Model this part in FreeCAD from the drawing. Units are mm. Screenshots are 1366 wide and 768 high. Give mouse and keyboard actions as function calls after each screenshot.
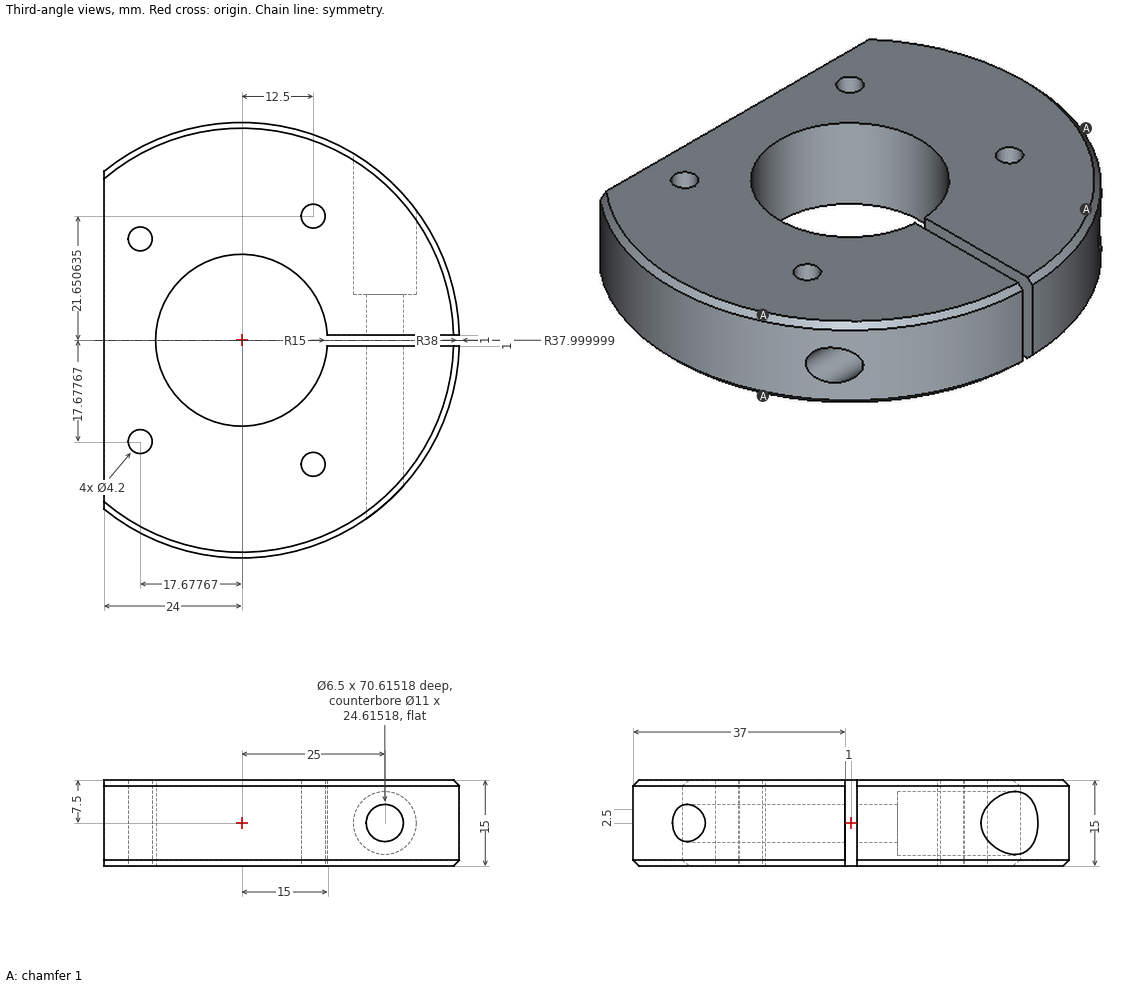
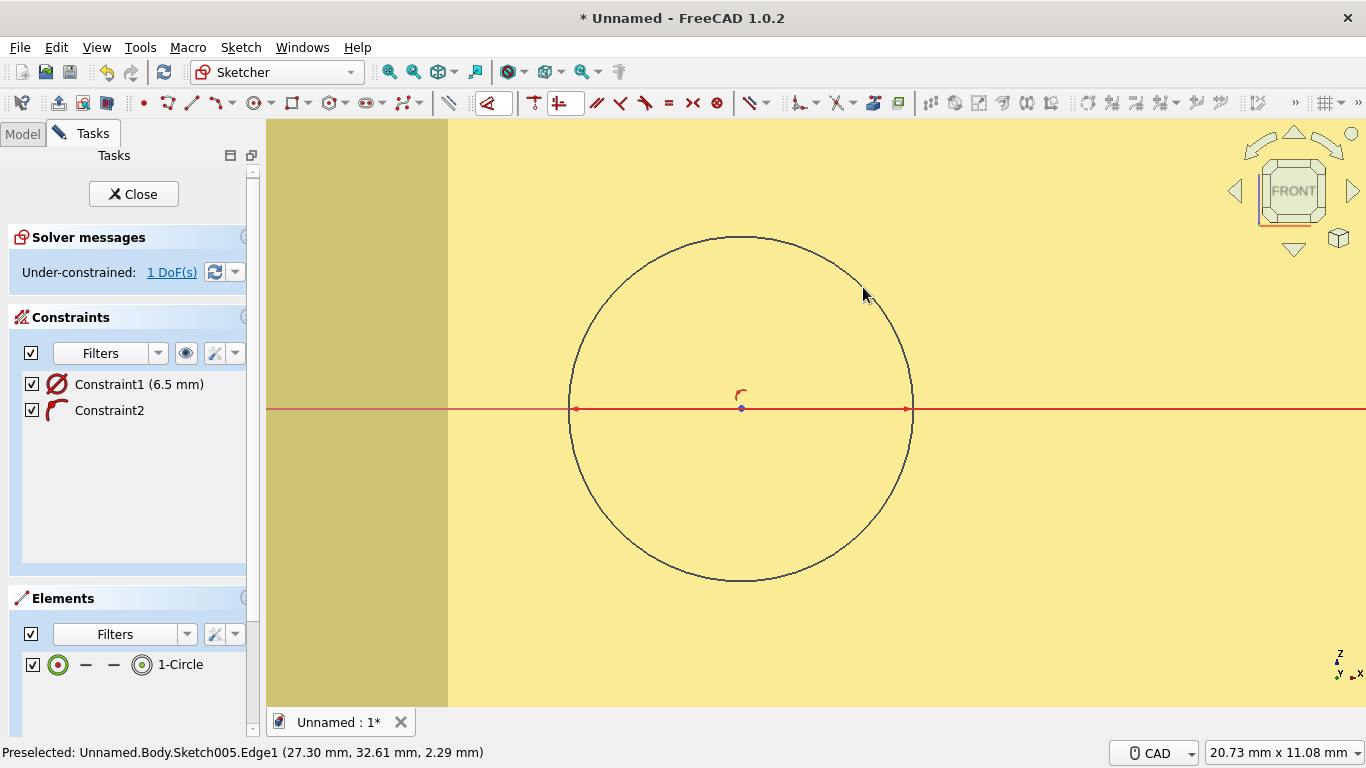
click(741, 409)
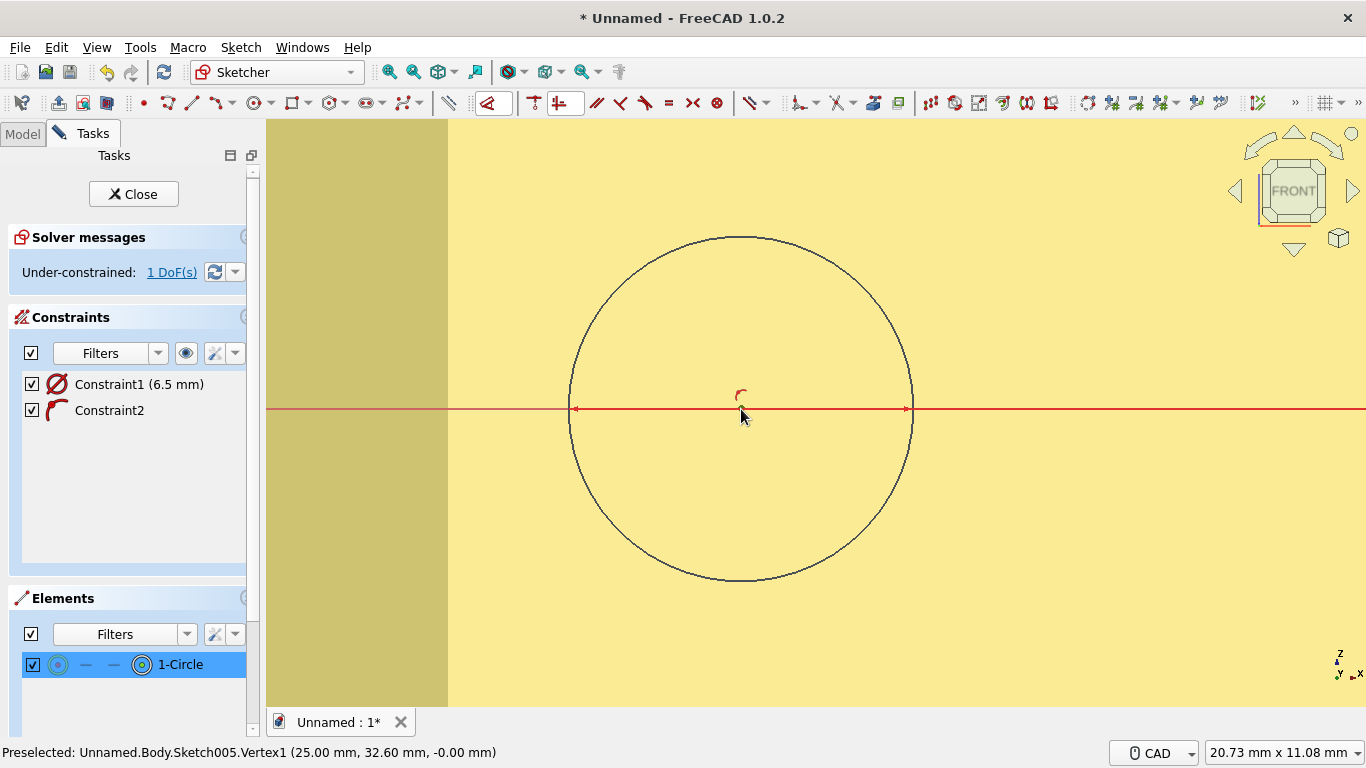
key(l)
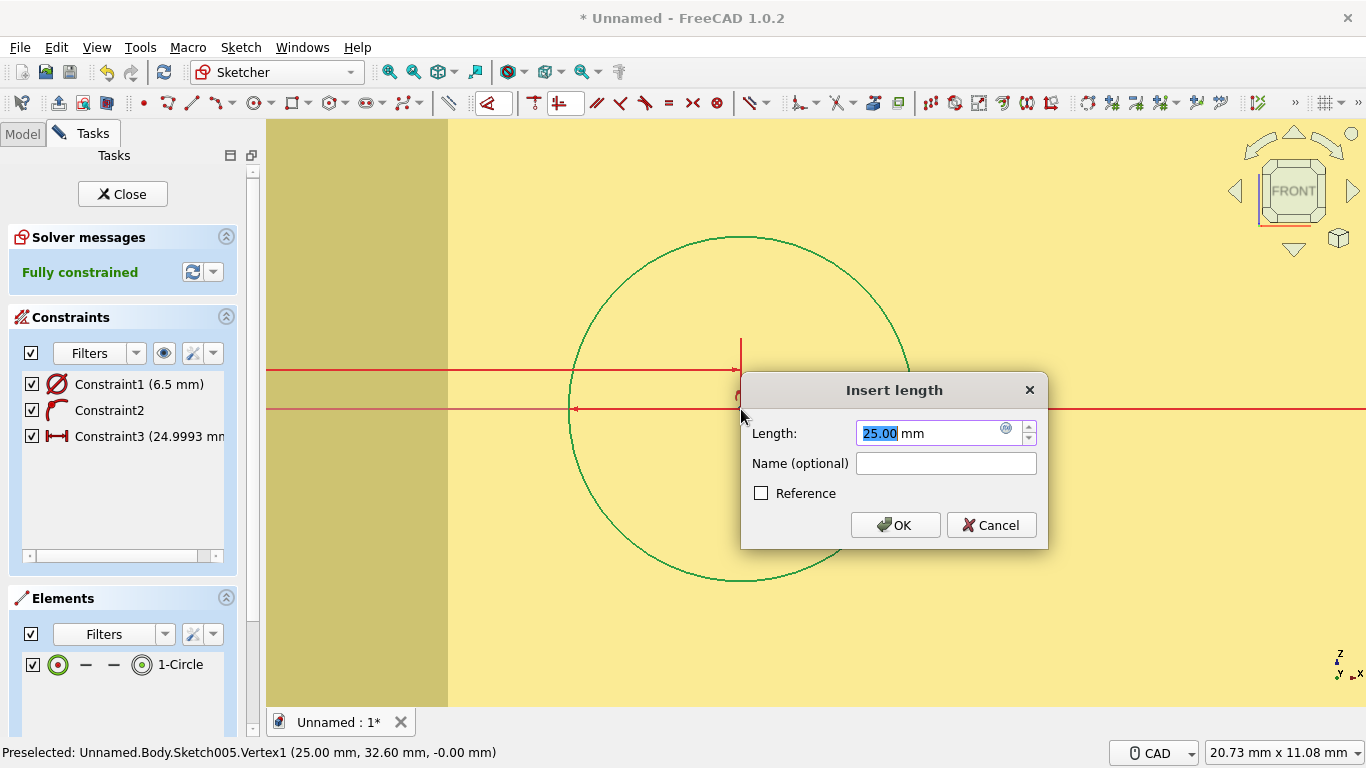
text(25)
key(Return)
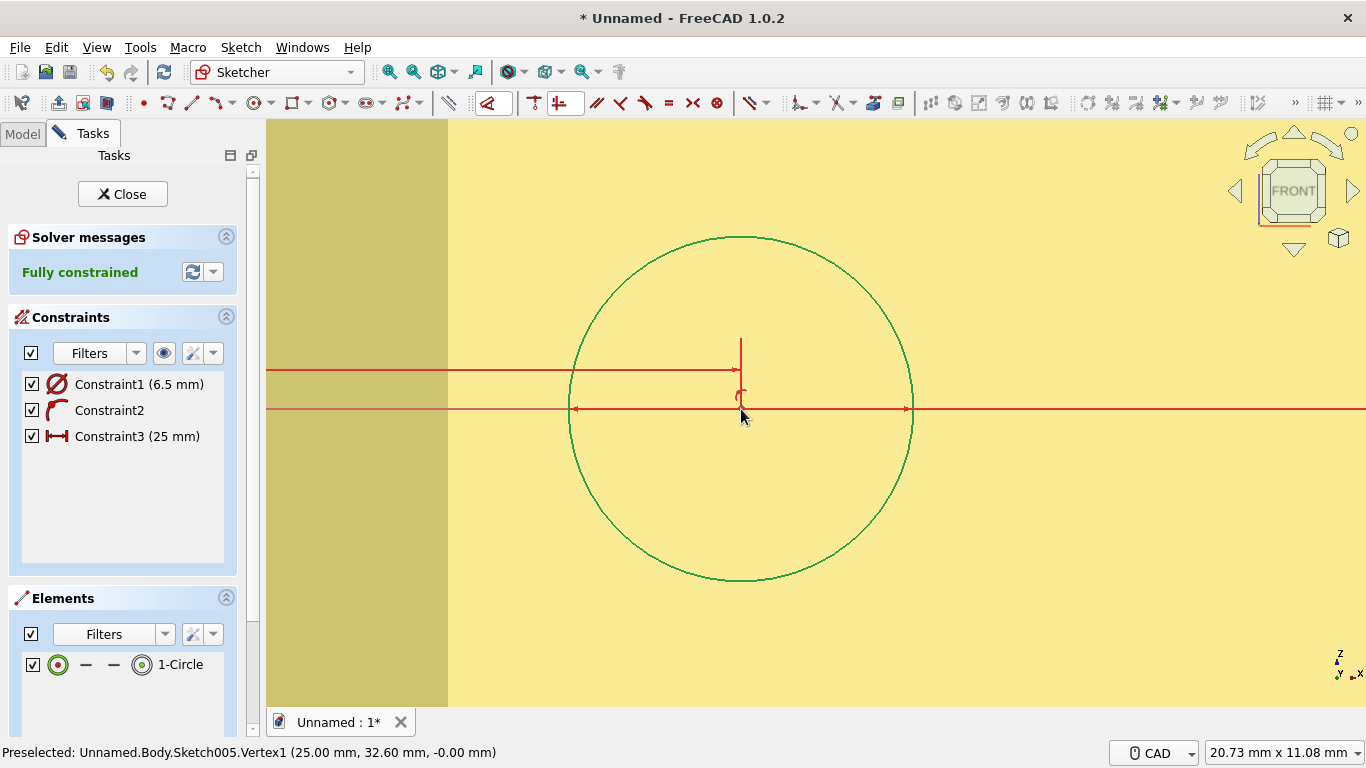
click(123, 194)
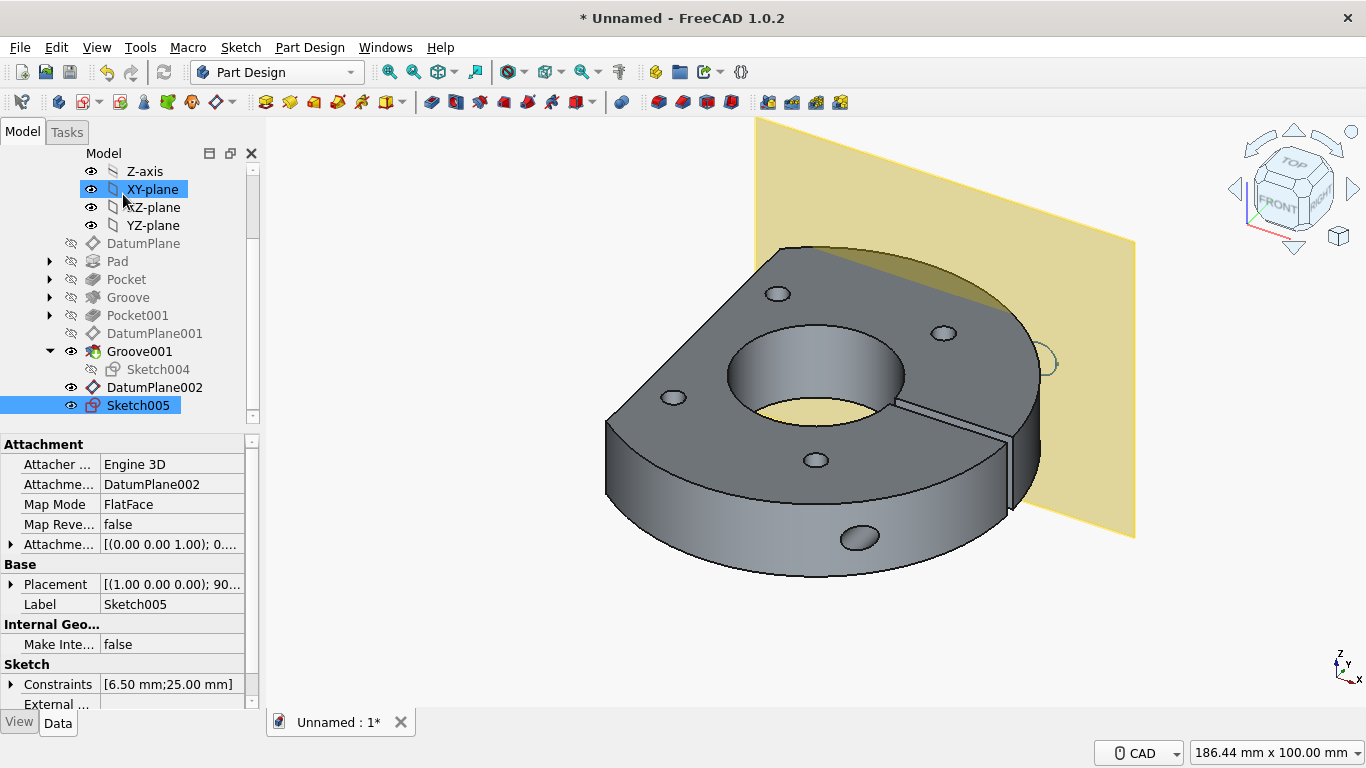
click(456, 102)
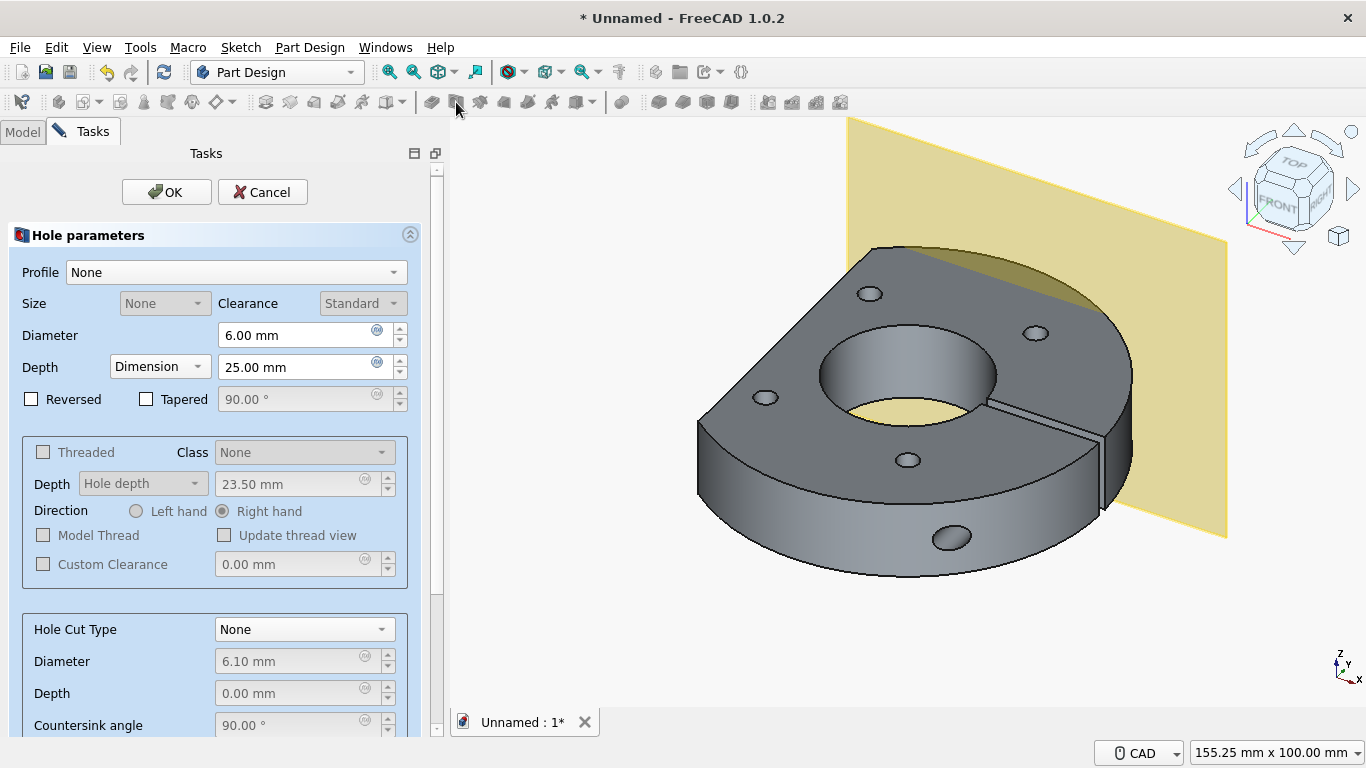
triple_click(305, 335)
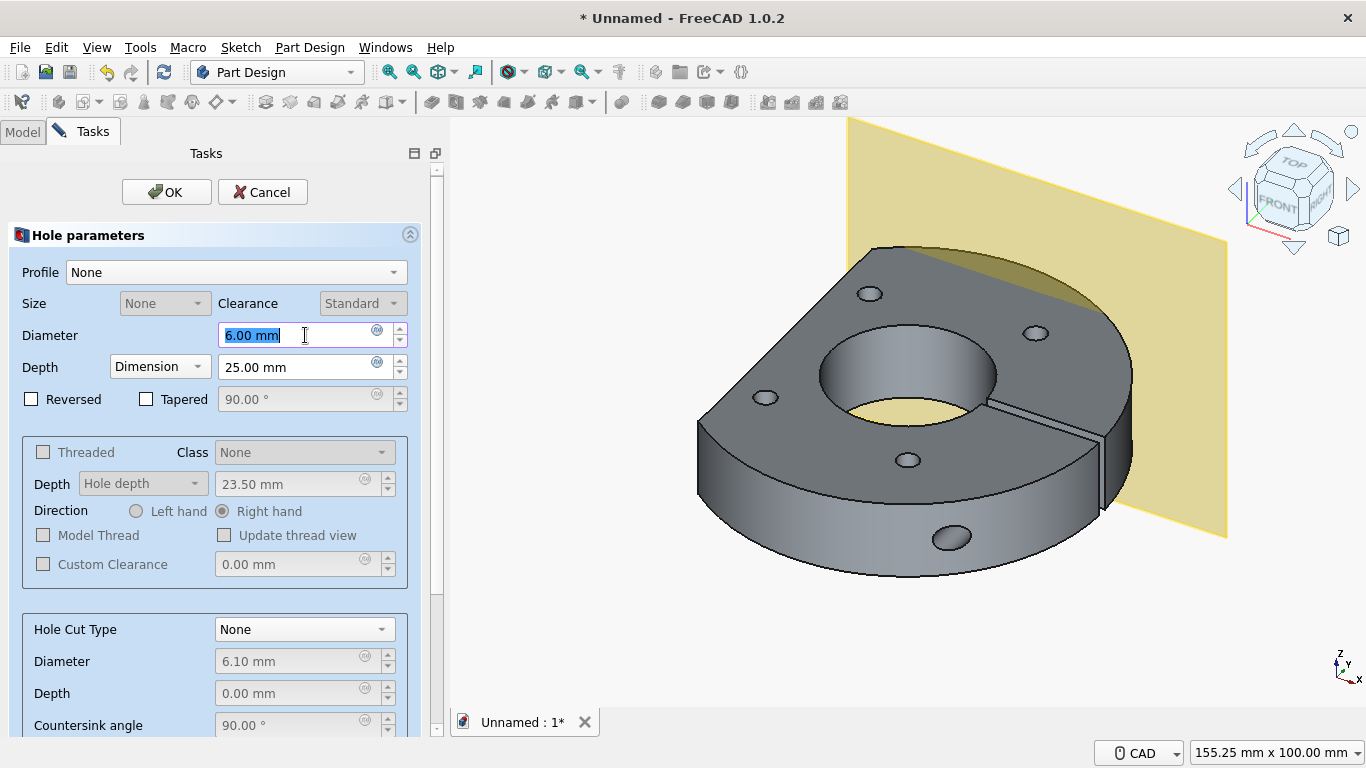
text(6.5)
key(Tab)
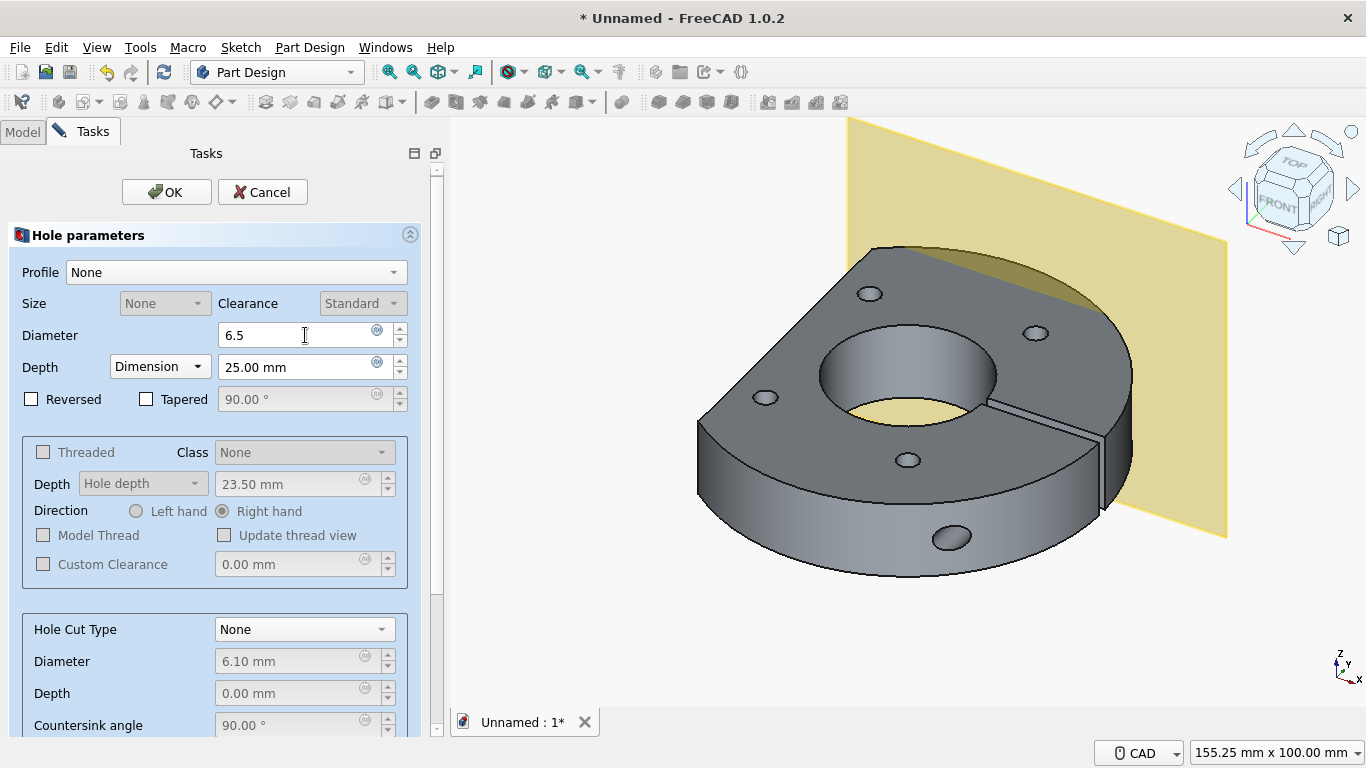
triple_click(305, 367)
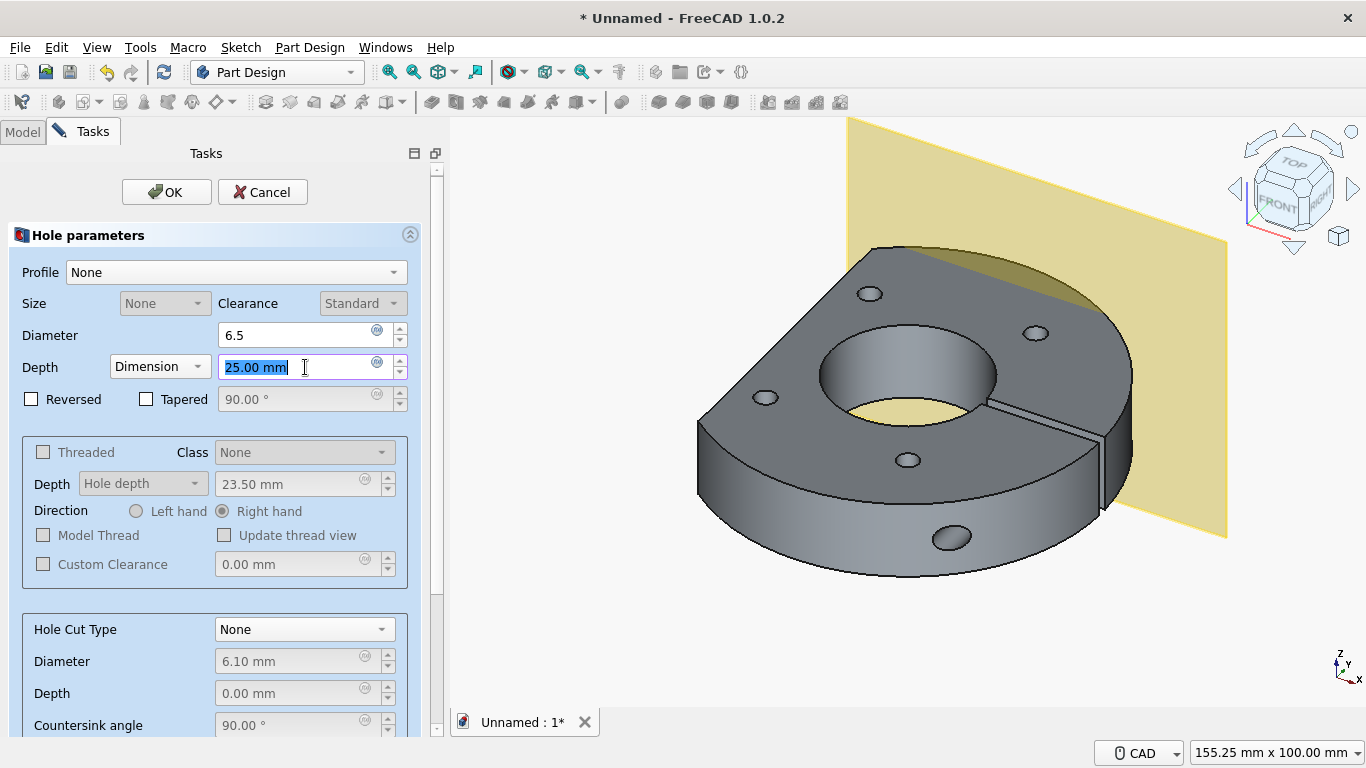
text(70.61518)
key(Tab)